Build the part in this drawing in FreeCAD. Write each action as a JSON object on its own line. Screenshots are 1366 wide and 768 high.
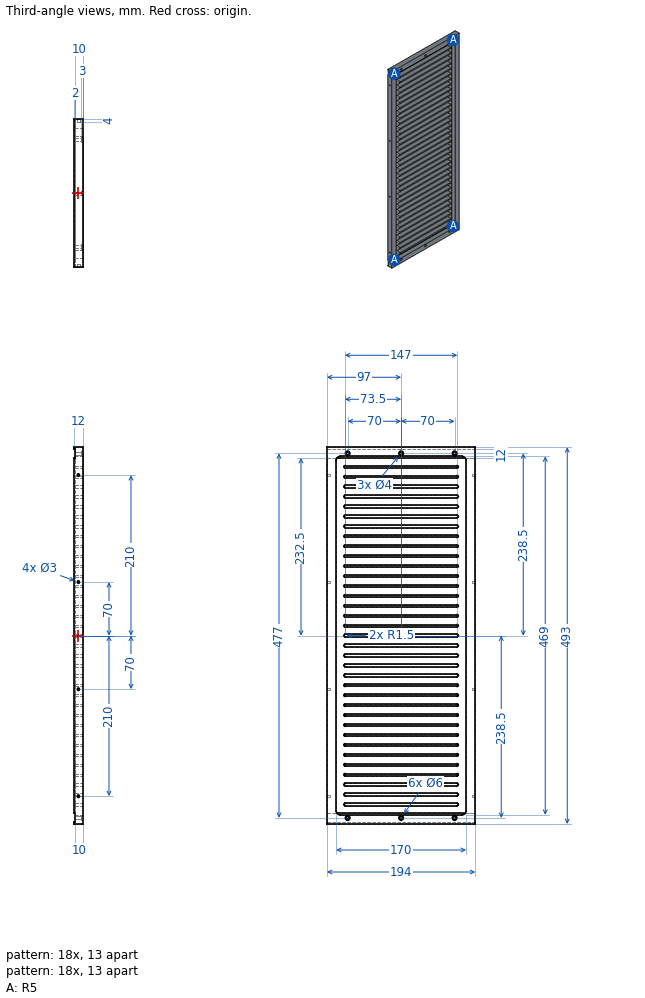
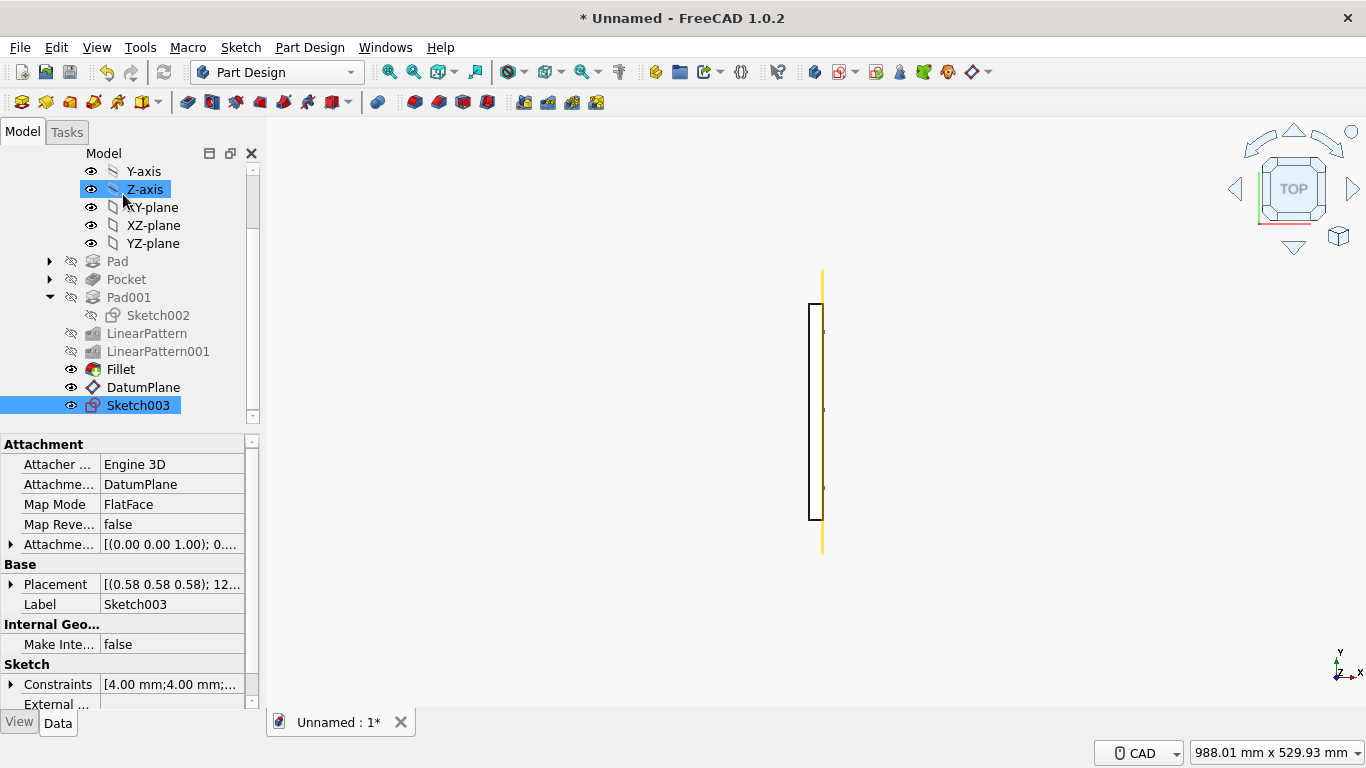
{"action": "left_click", "coordinate": [188, 102]}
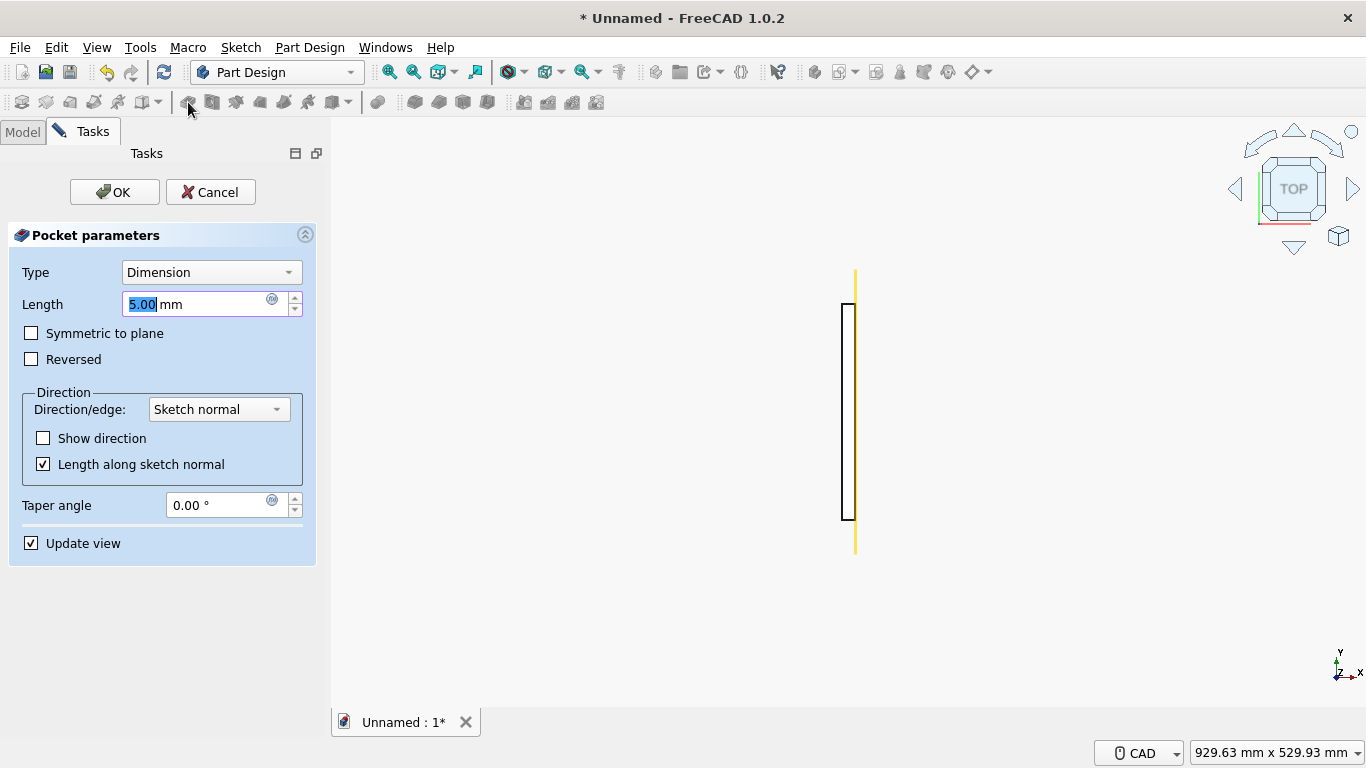
{"action": "left_click", "coordinate": [212, 272]}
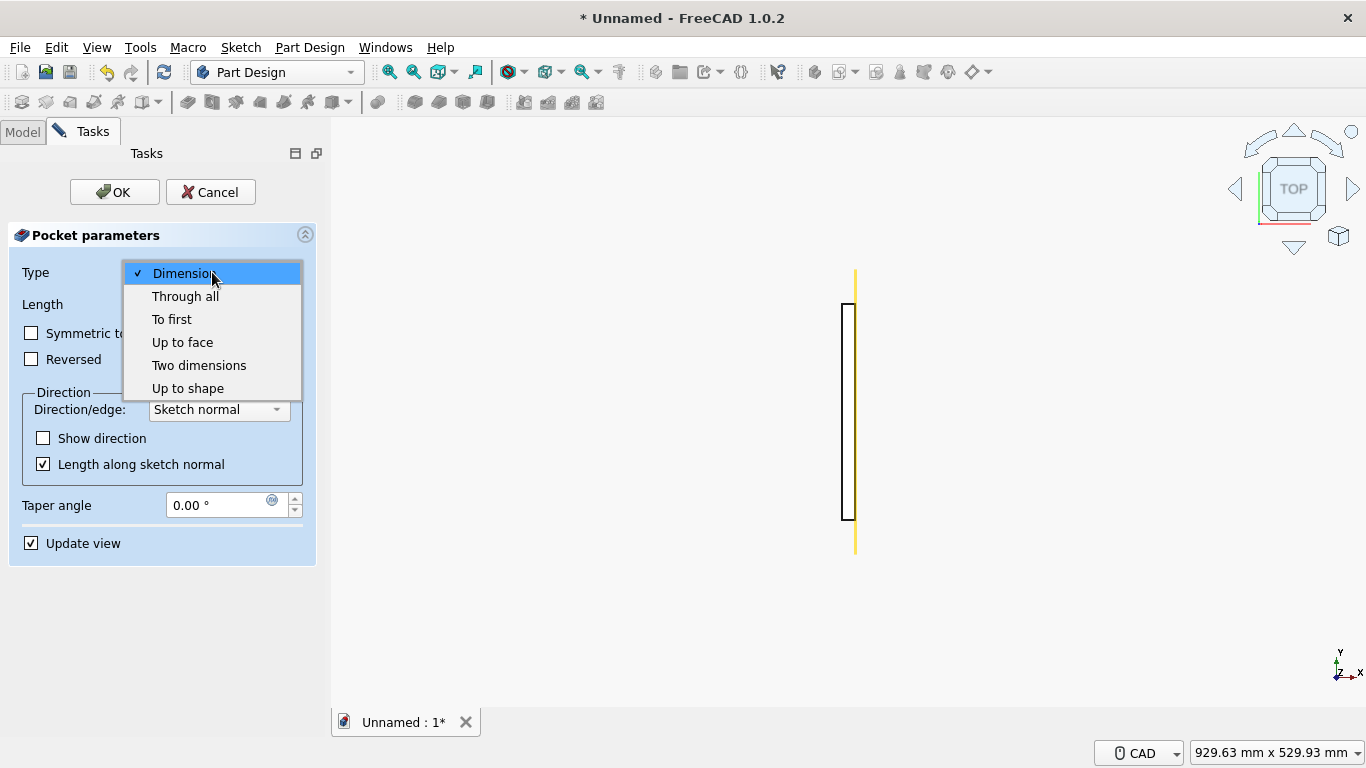
{"action": "left_click", "coordinate": [212, 296]}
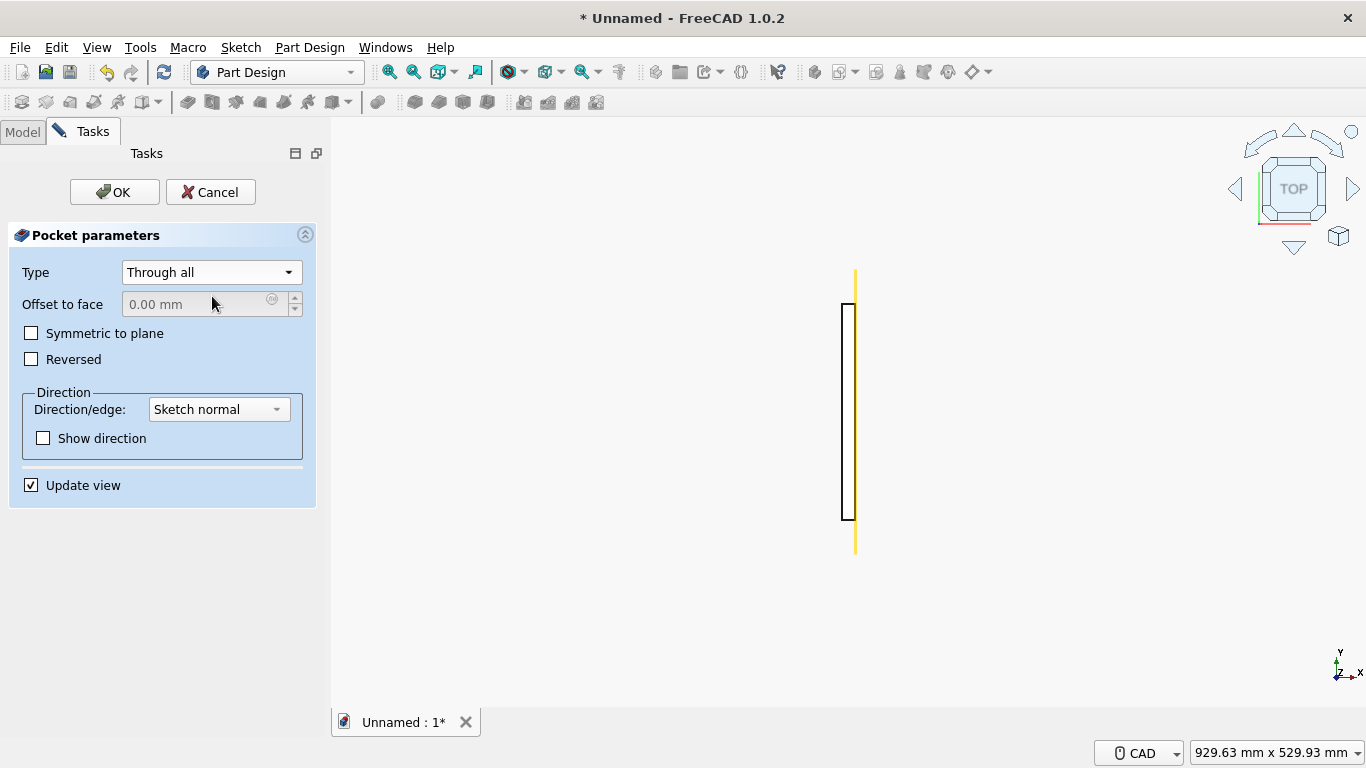
{"action": "left_click", "coordinate": [115, 192]}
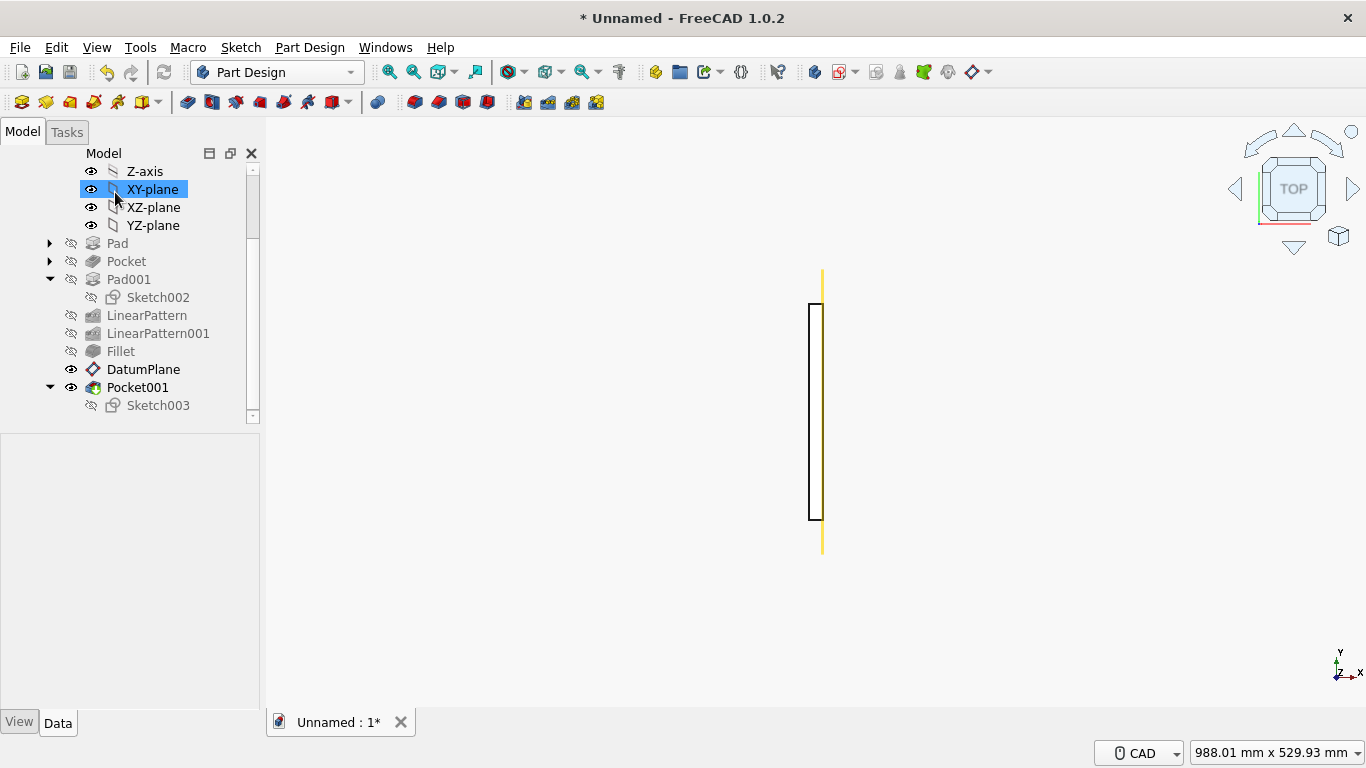
{"action": "left_click", "coordinate": [116, 369]}
{"action": "key", "text": "space"}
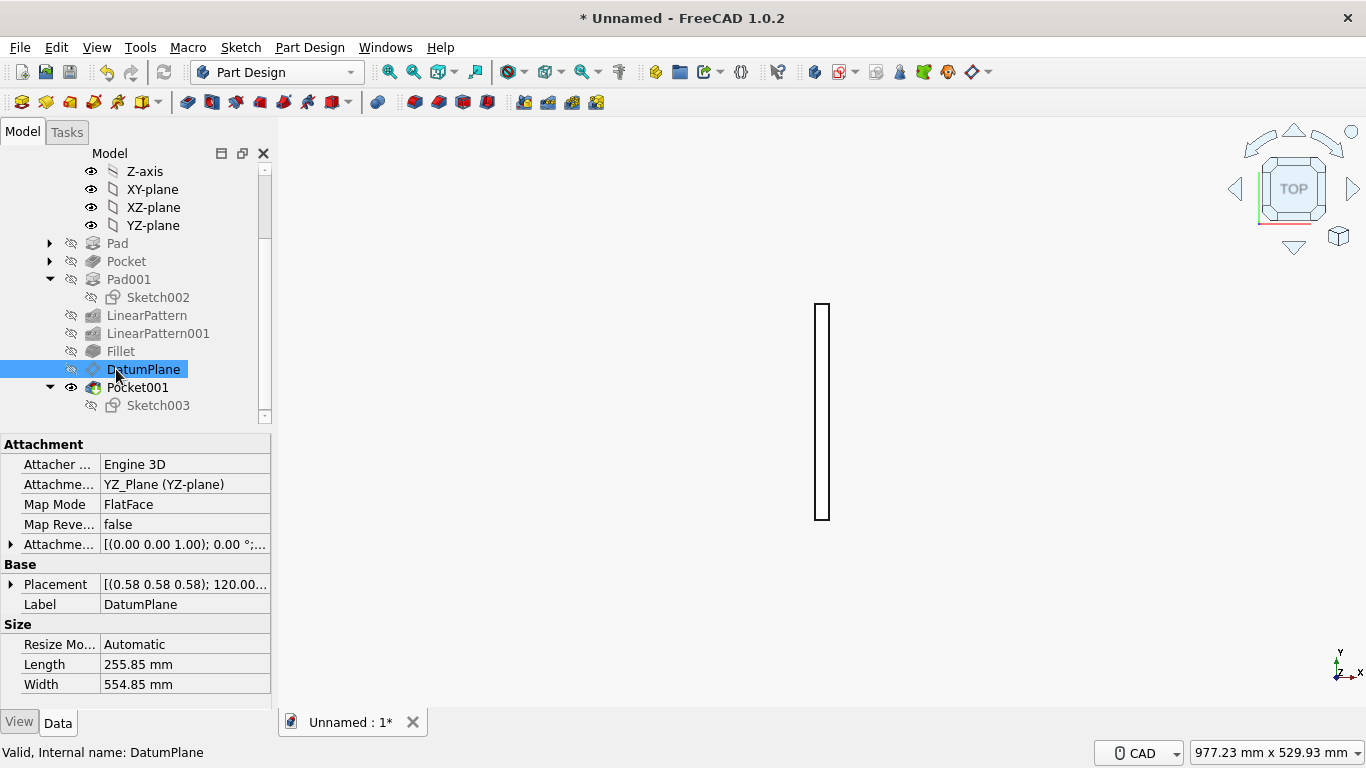
{"action": "left_click", "coordinate": [390, 72]}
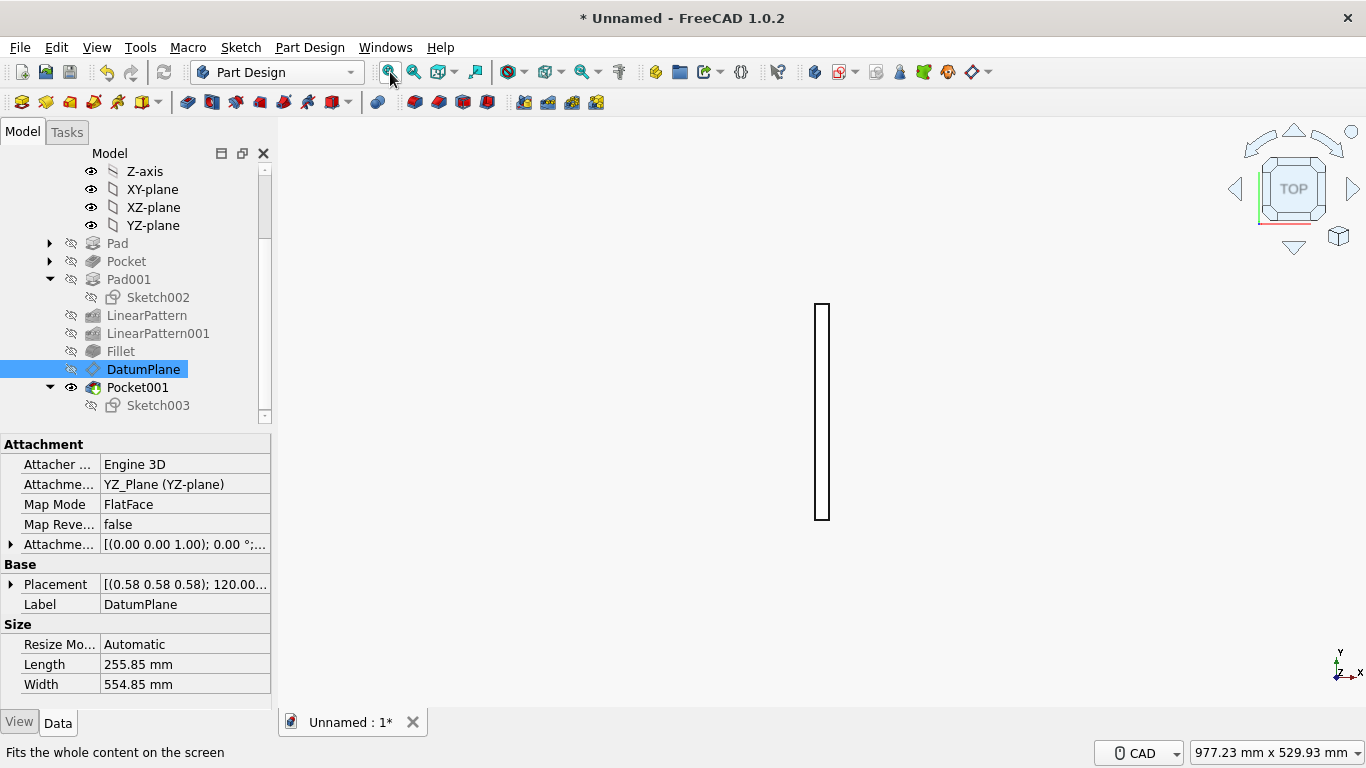
{"action": "left_click", "coordinate": [116, 387]}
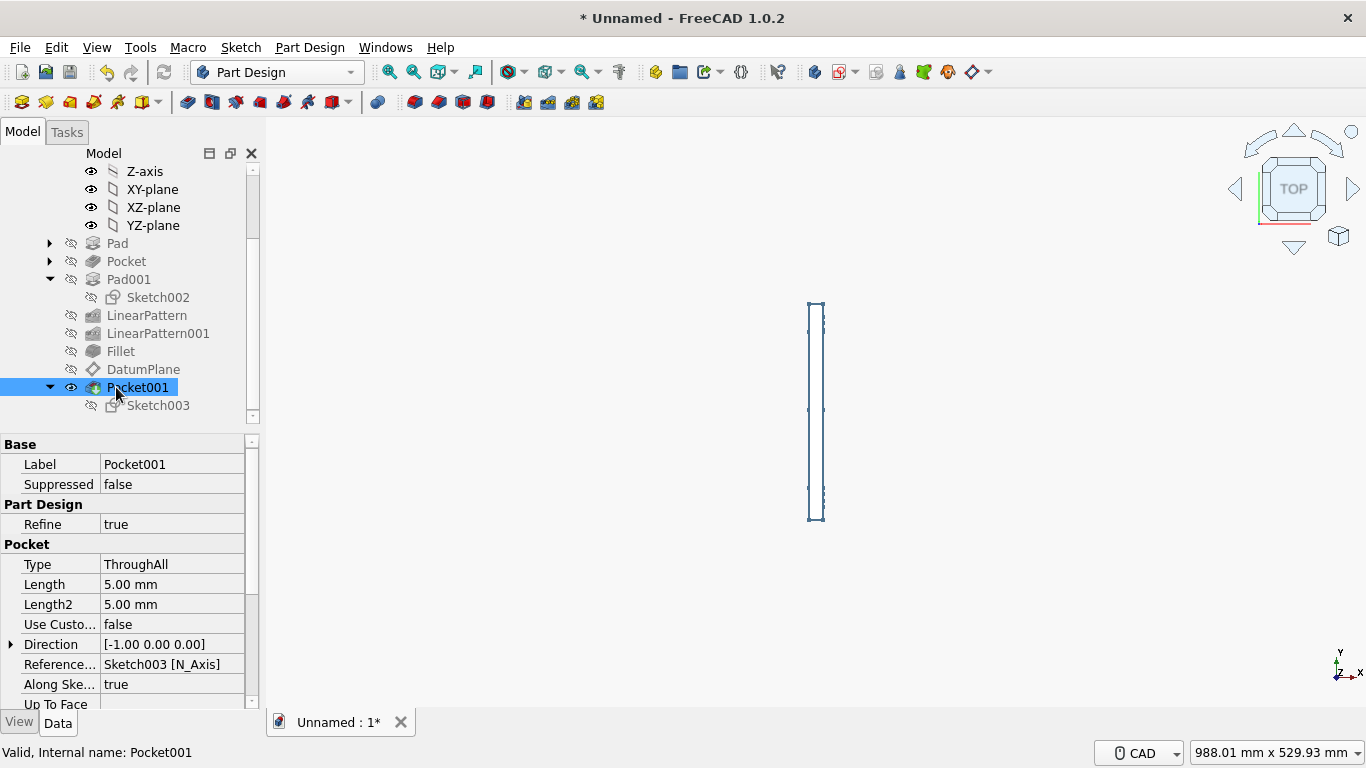
{"action": "left_click", "coordinate": [524, 102]}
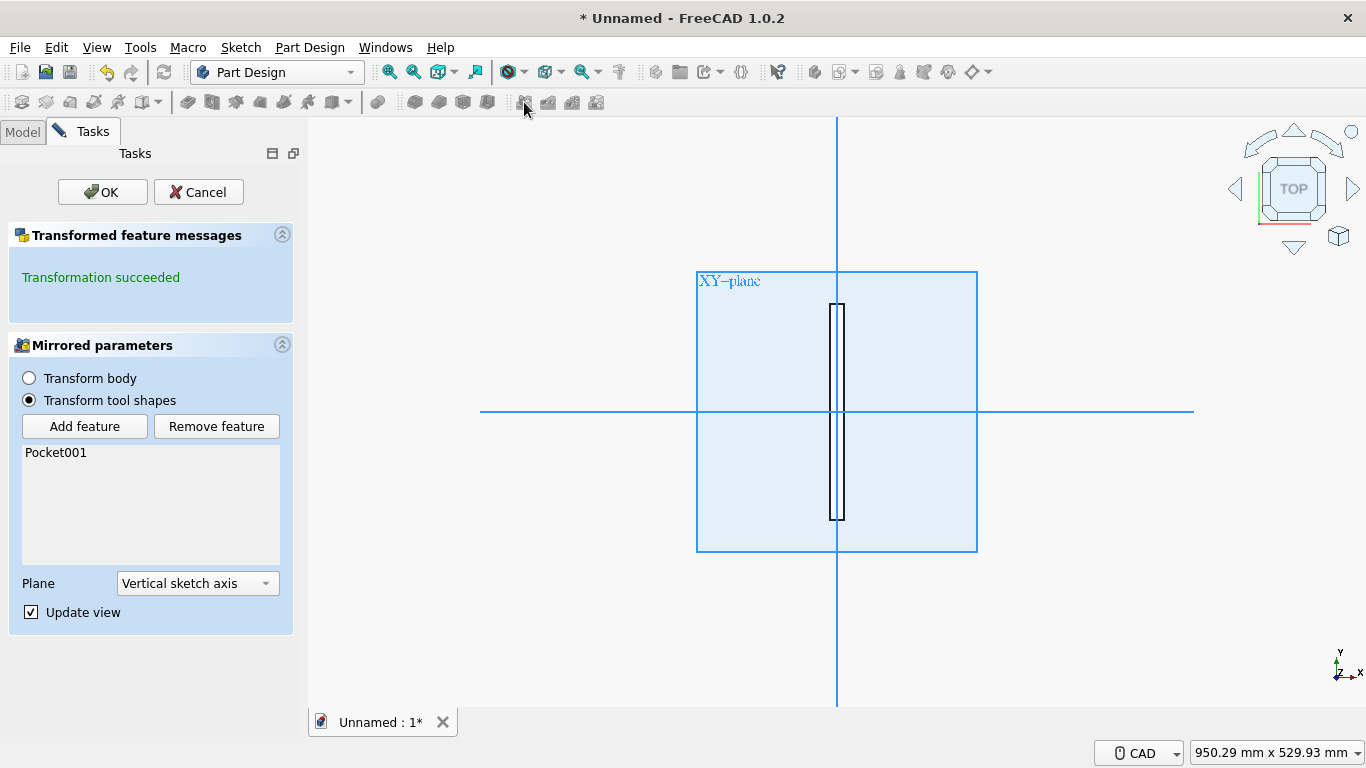
{"action": "left_click", "coordinate": [198, 584]}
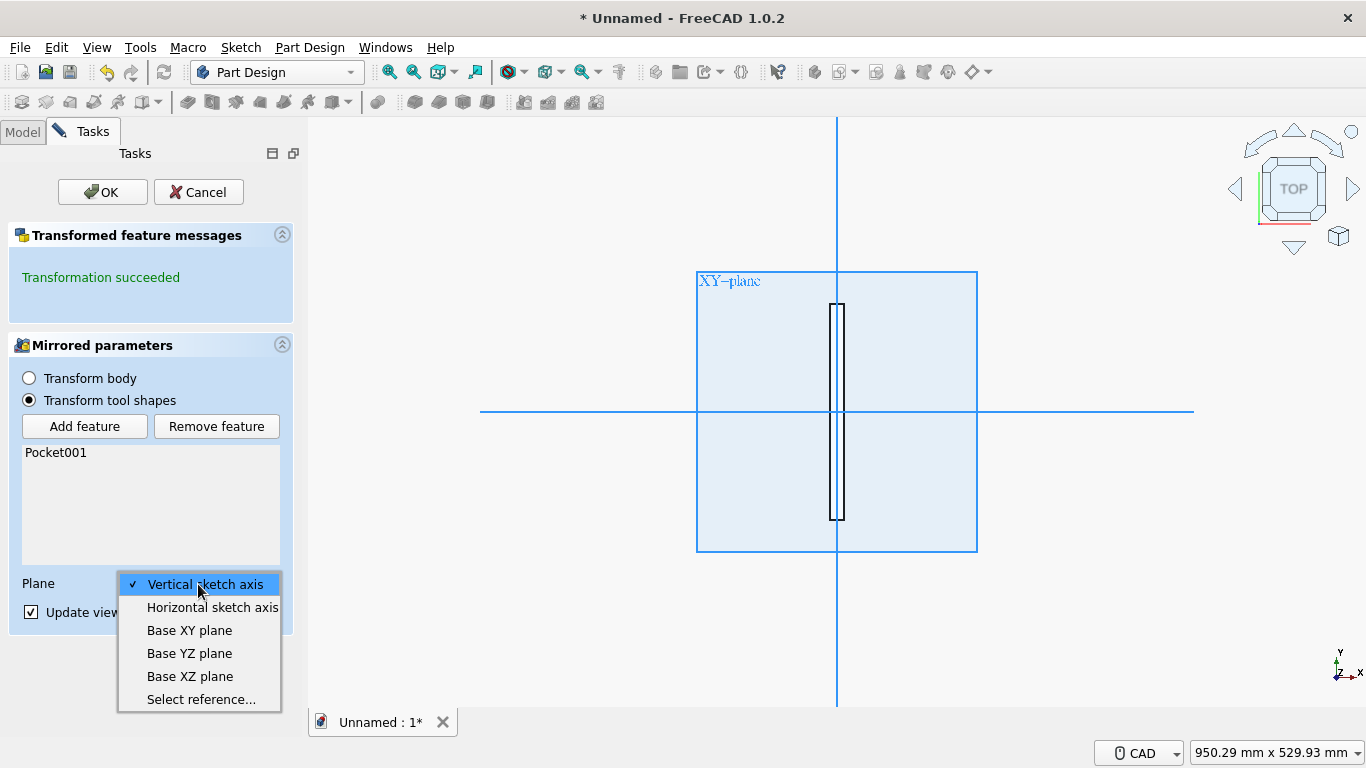
{"action": "left_click", "coordinate": [198, 630]}